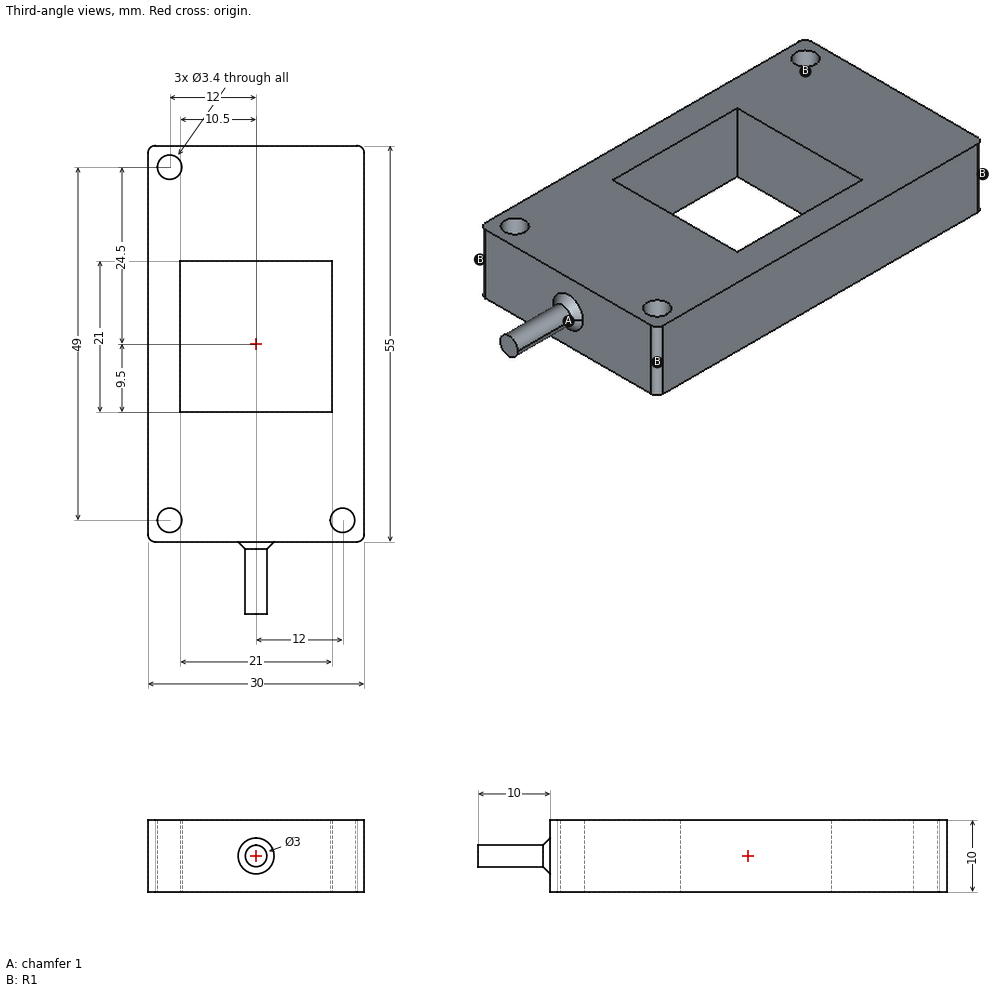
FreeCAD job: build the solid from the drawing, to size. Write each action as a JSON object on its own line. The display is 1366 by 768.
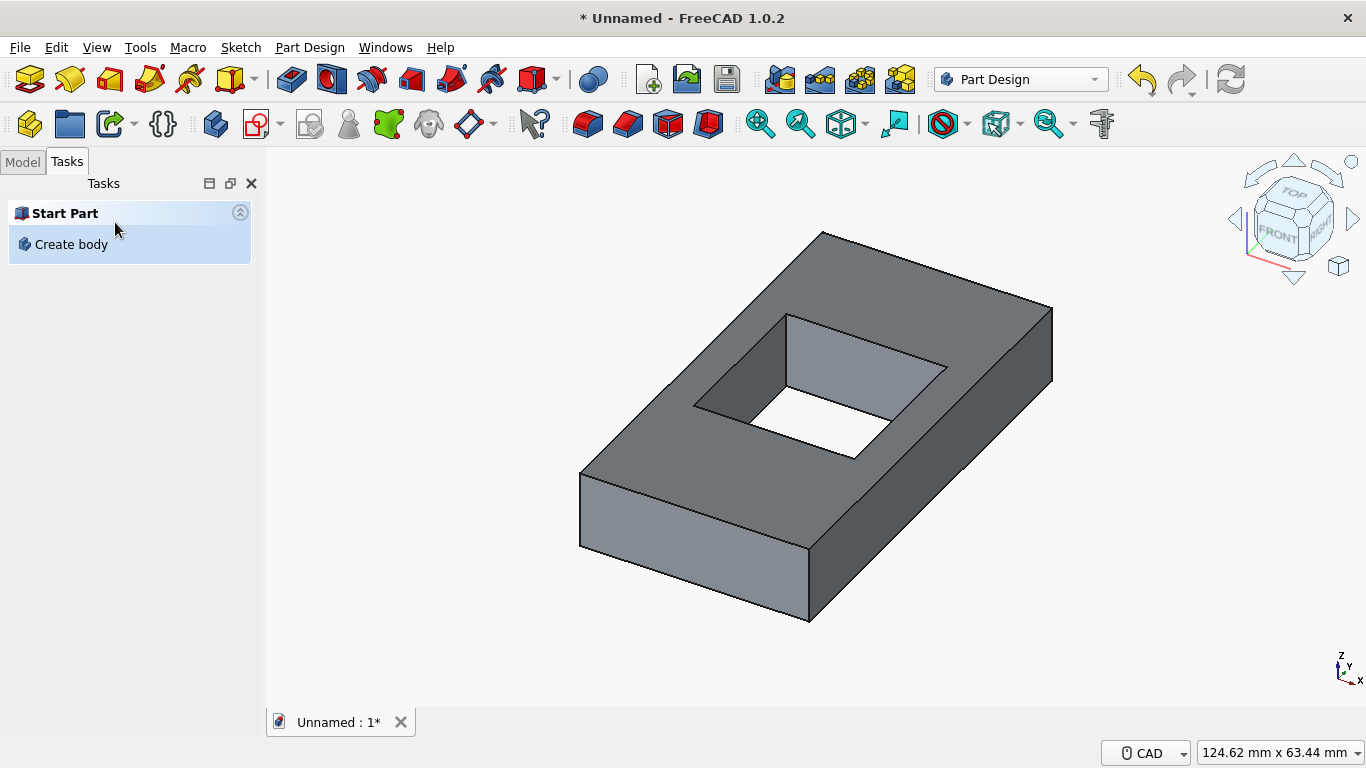
{"action": "left_click", "coordinate": [760, 568]}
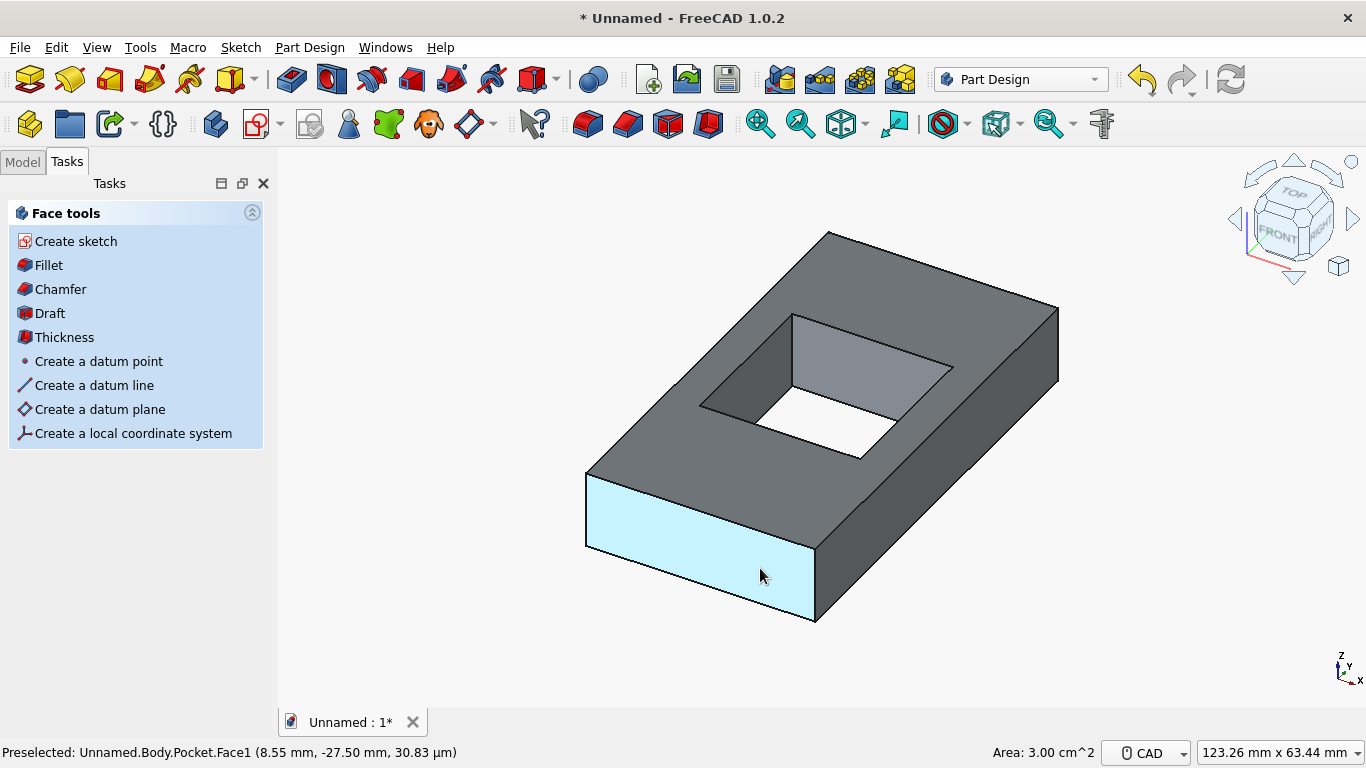
{"action": "left_click", "coordinate": [256, 124]}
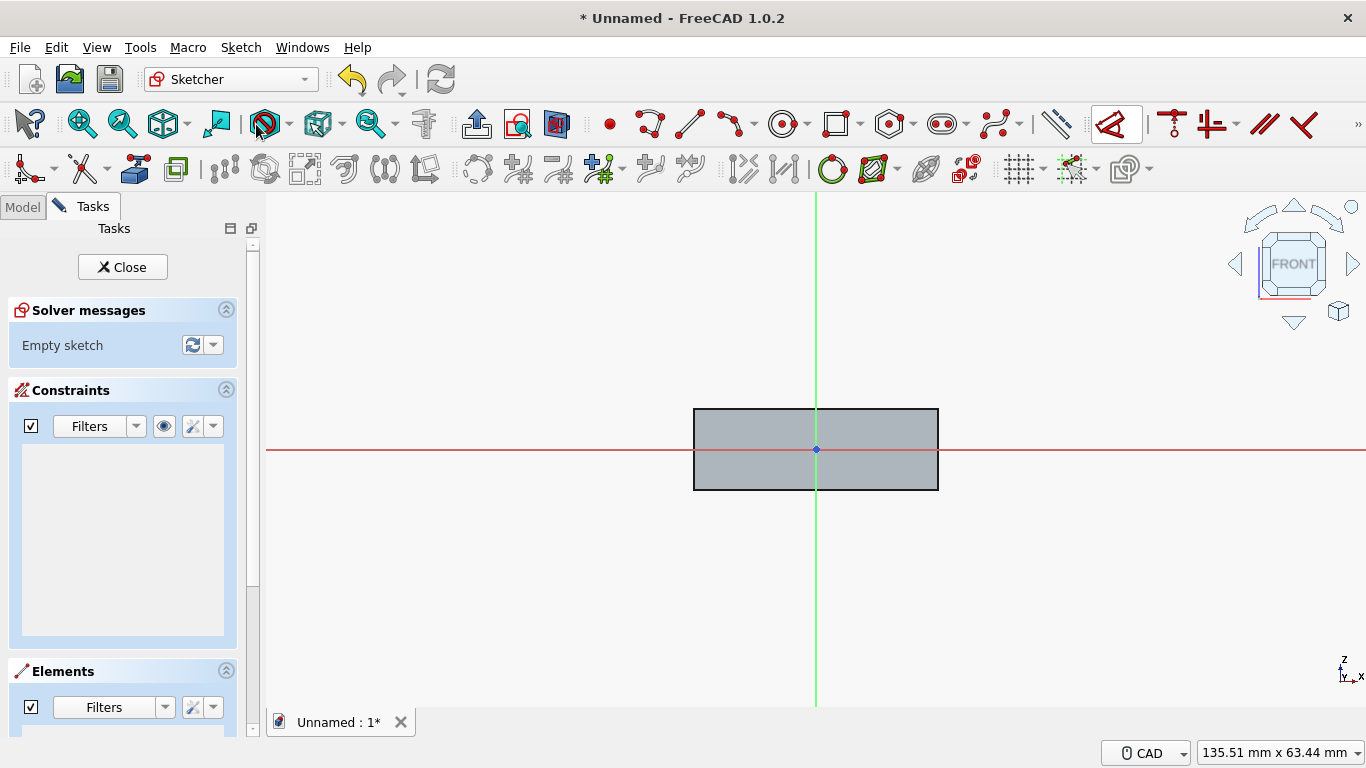
{"action": "scroll", "coordinate": [821, 450], "scroll_direction": "up", "scroll_amount": 13}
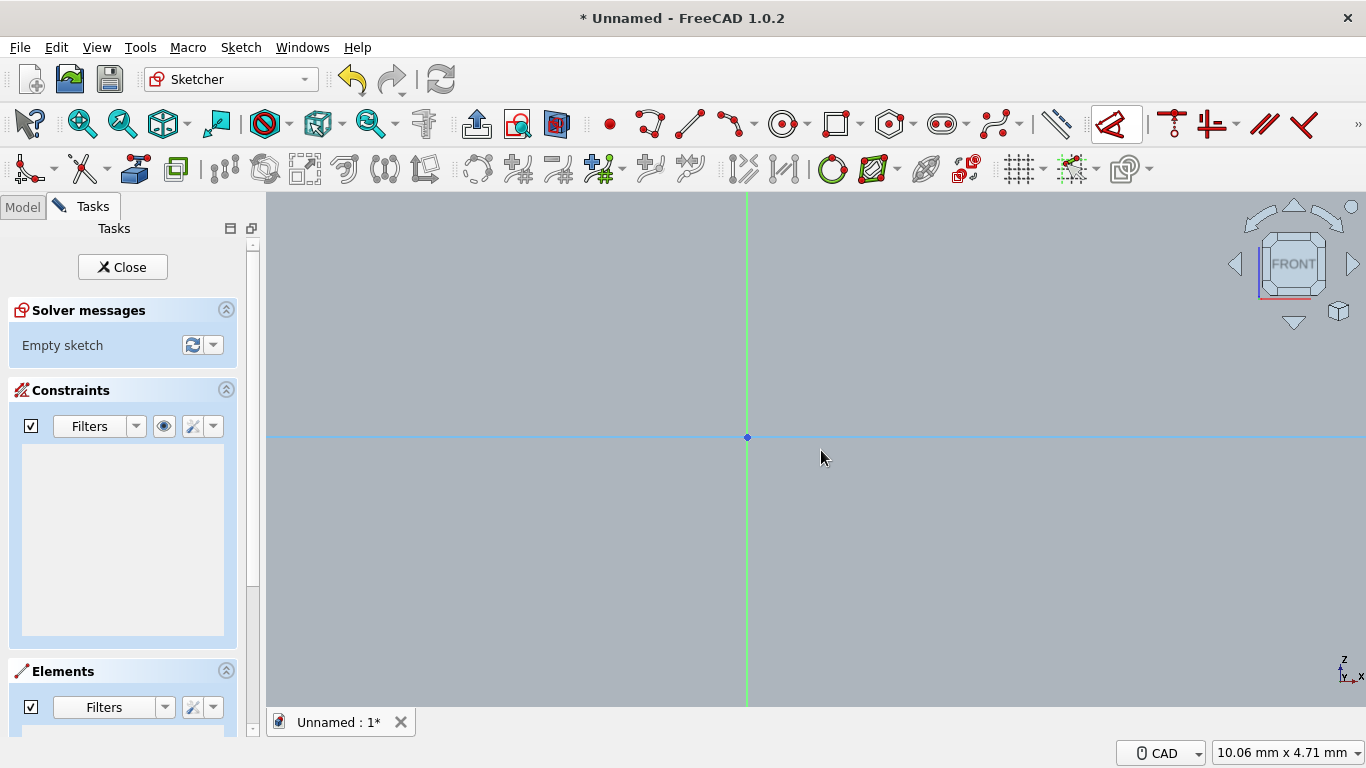
{"action": "key", "text": "g c"}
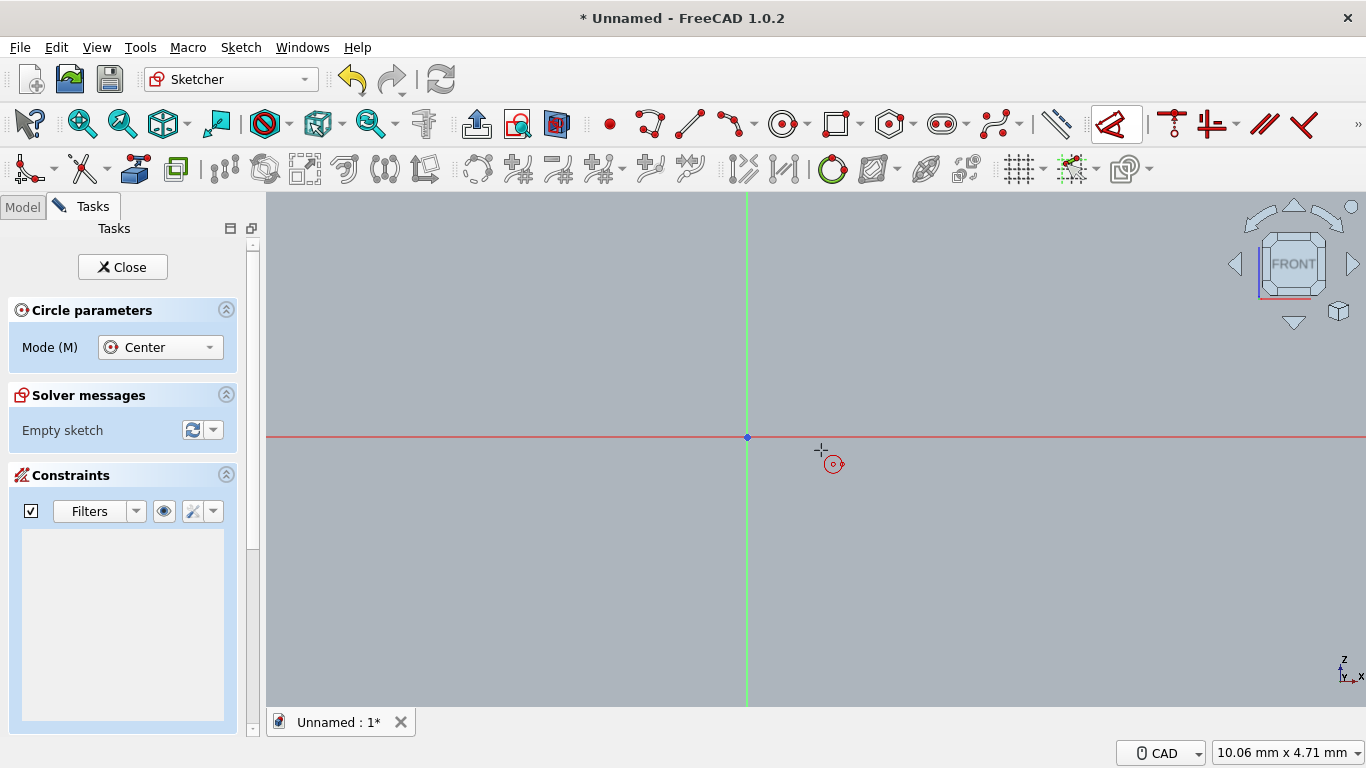
{"action": "left_click", "coordinate": [747, 437]}
{"action": "left_click", "coordinate": [863, 321]}
{"action": "key", "text": "Escape"}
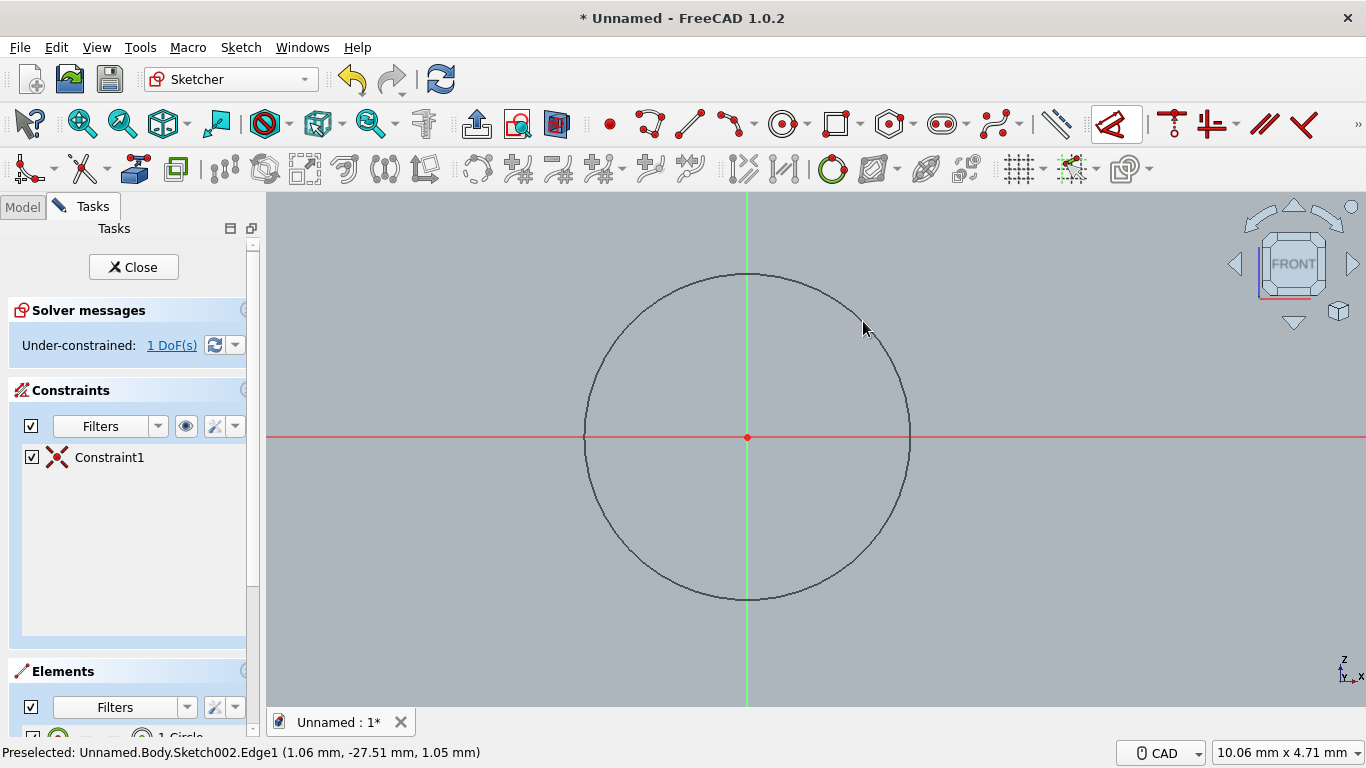
{"action": "key", "text": "d"}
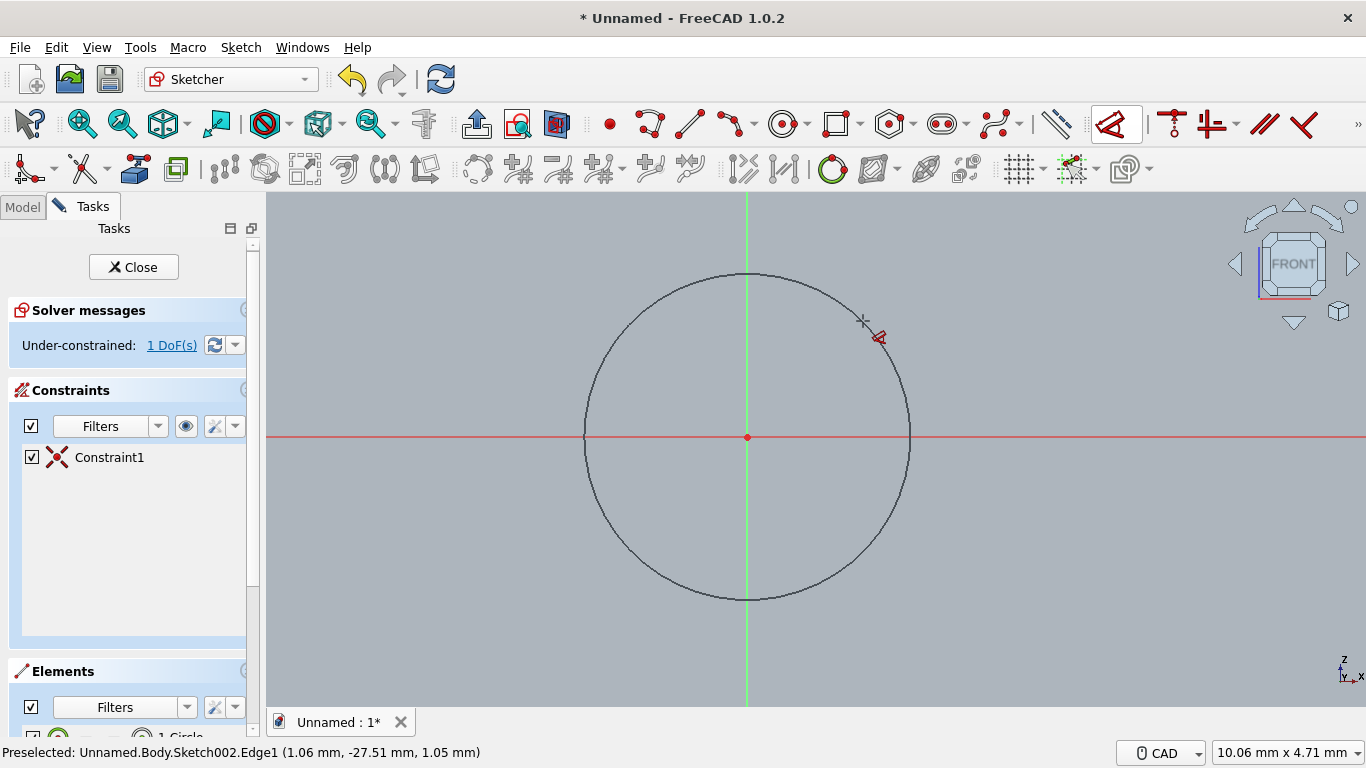
{"action": "left_click", "coordinate": [862, 321]}
{"action": "left_click", "coordinate": [884, 298]}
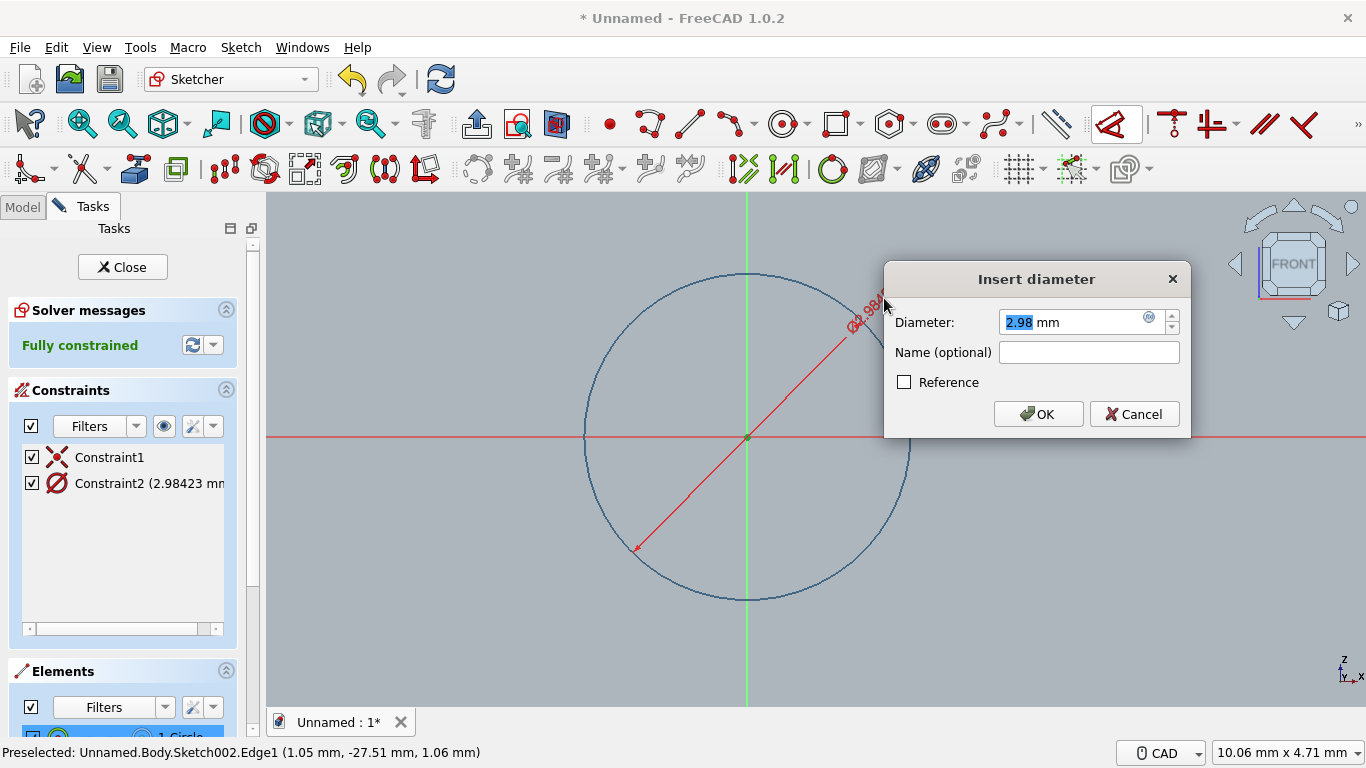
{"action": "type", "text": "3"}
{"action": "key", "text": "Return"}
{"action": "key", "text": "Escape"}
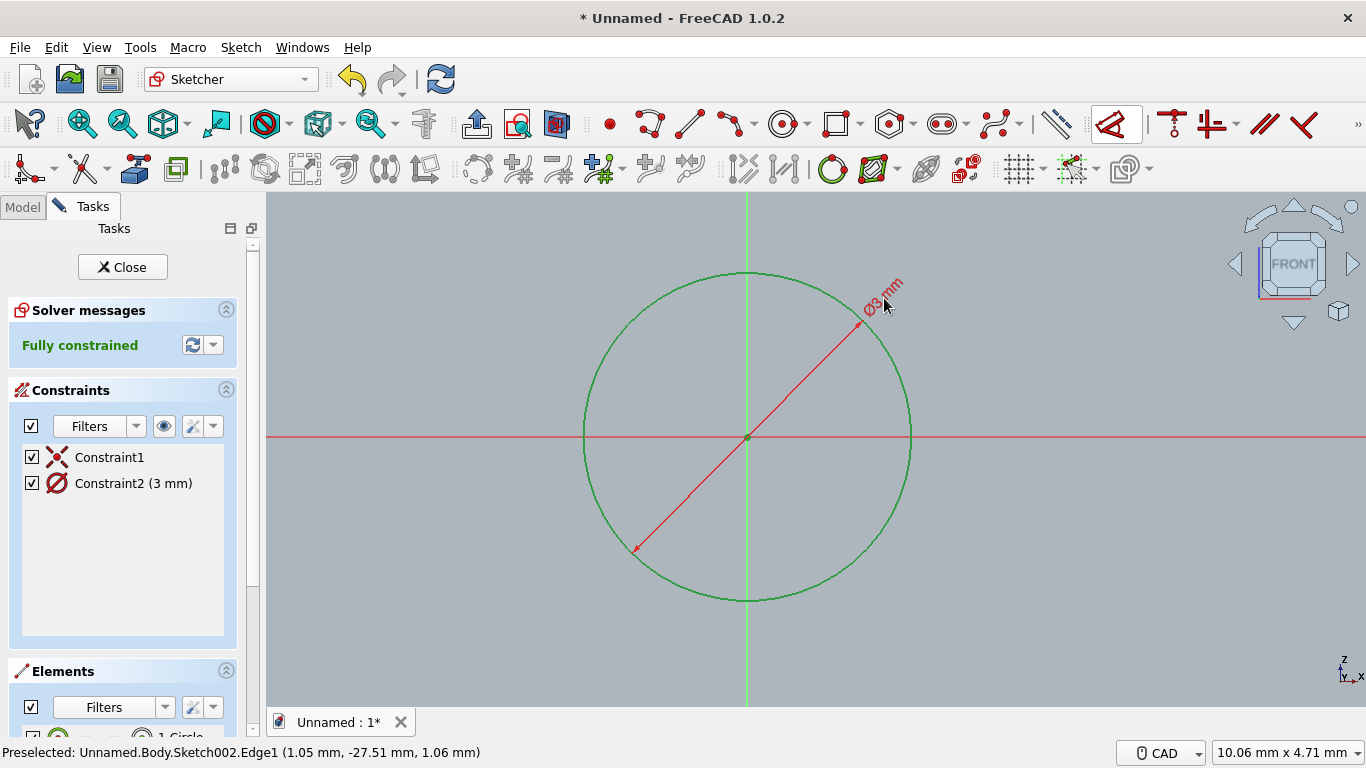
{"action": "left_click", "coordinate": [123, 267]}